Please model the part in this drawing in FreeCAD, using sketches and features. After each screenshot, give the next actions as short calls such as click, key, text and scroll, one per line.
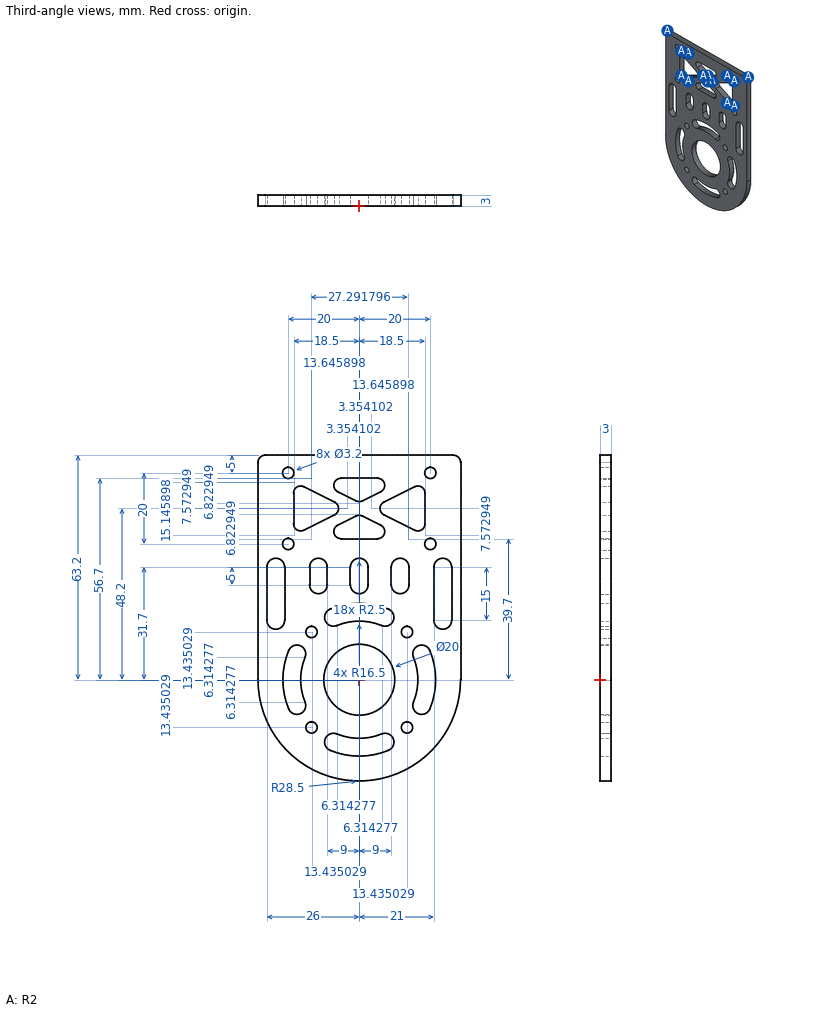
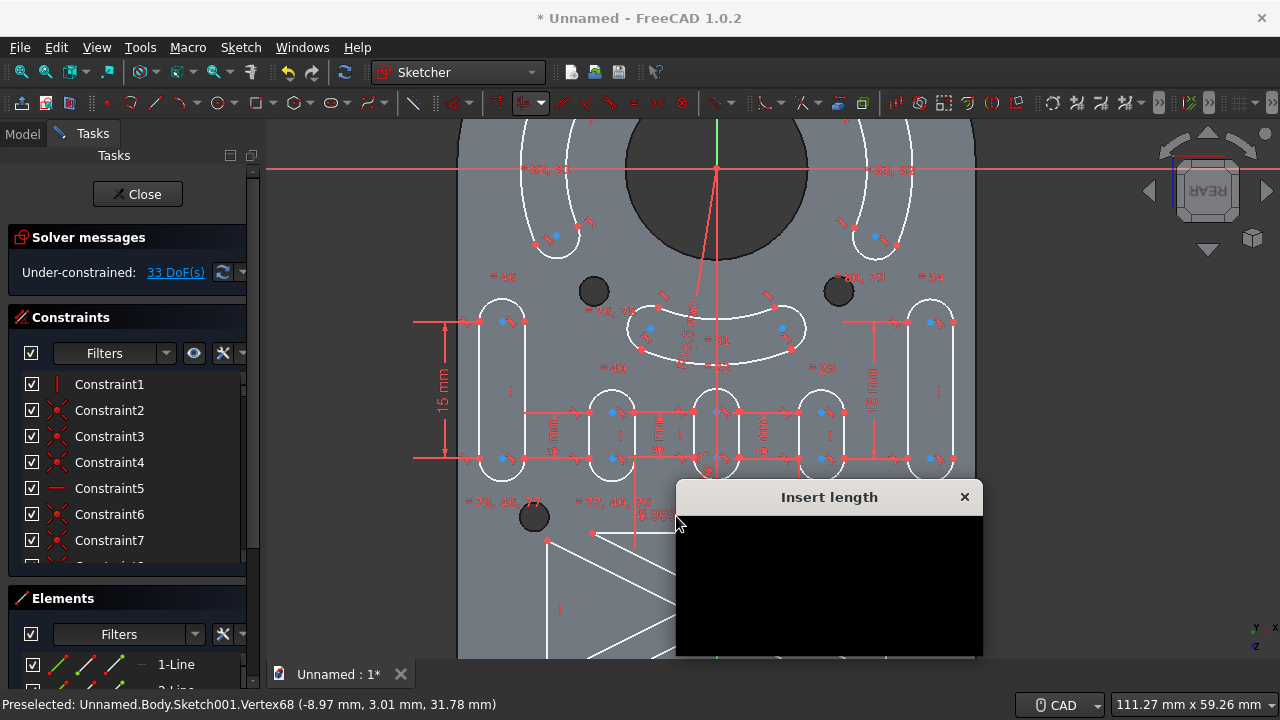
text(9)
key(Return)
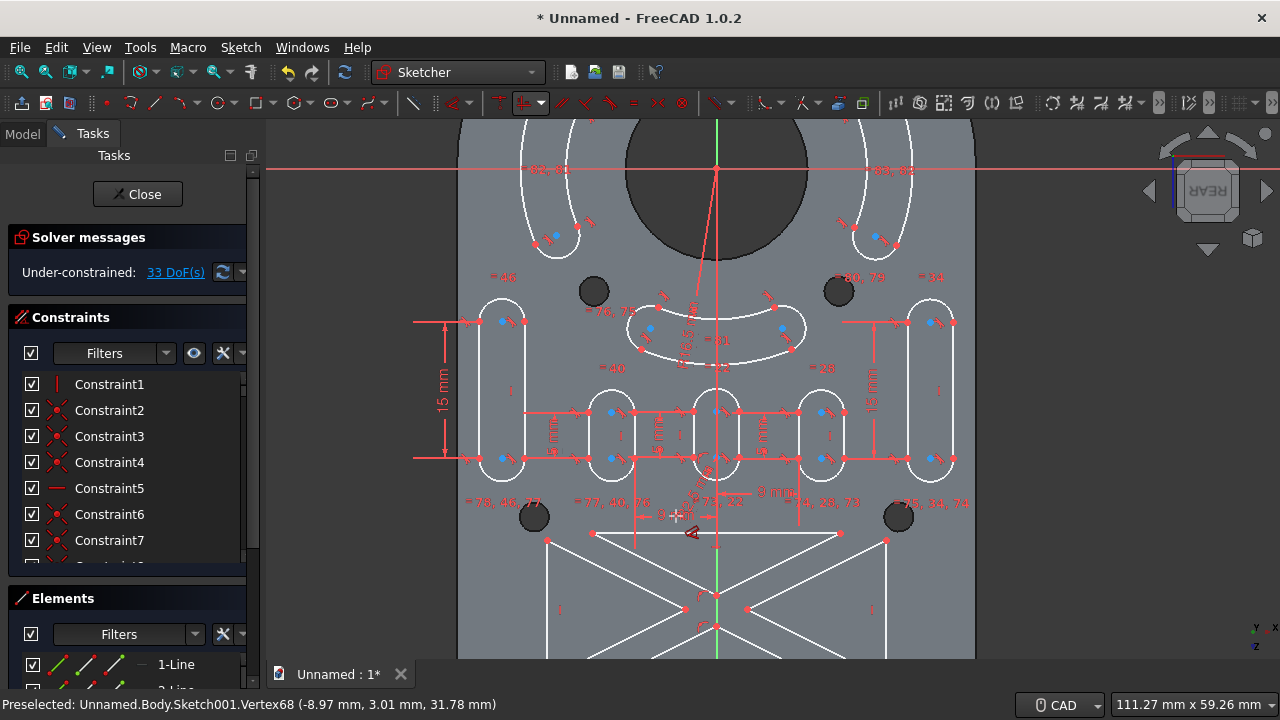
click(908, 459)
click(856, 493)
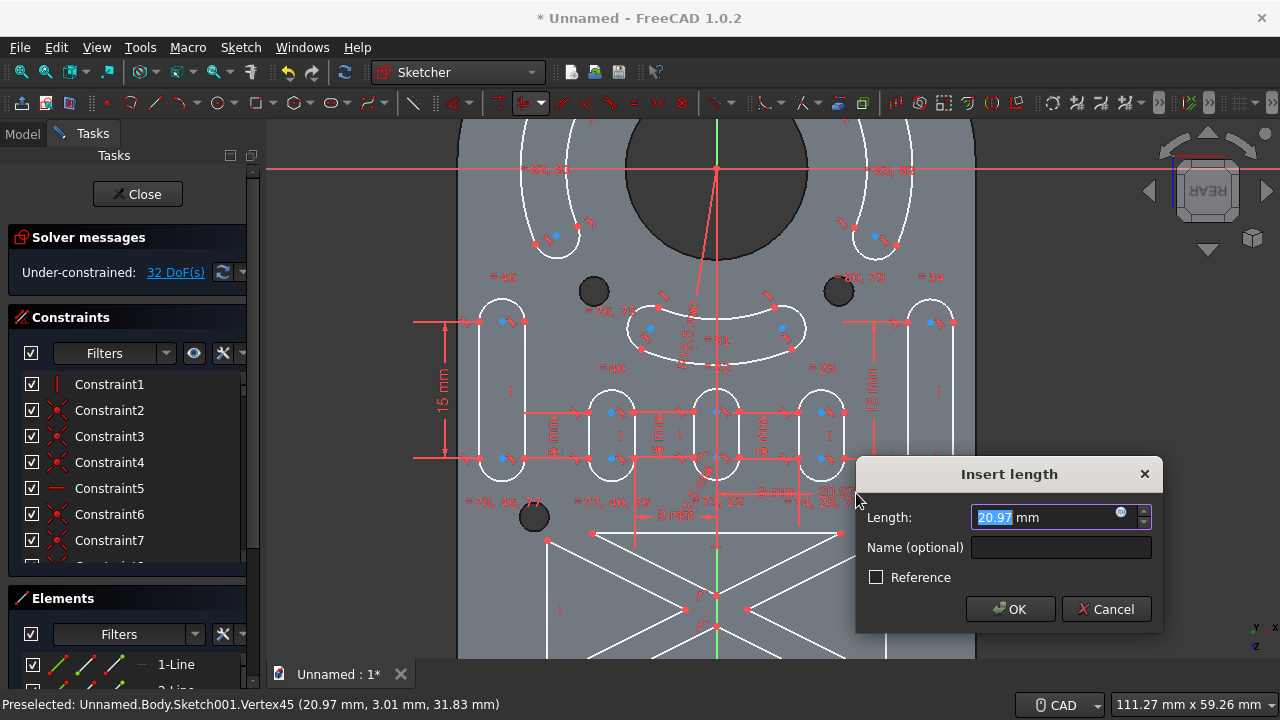
text(21)
key(Return)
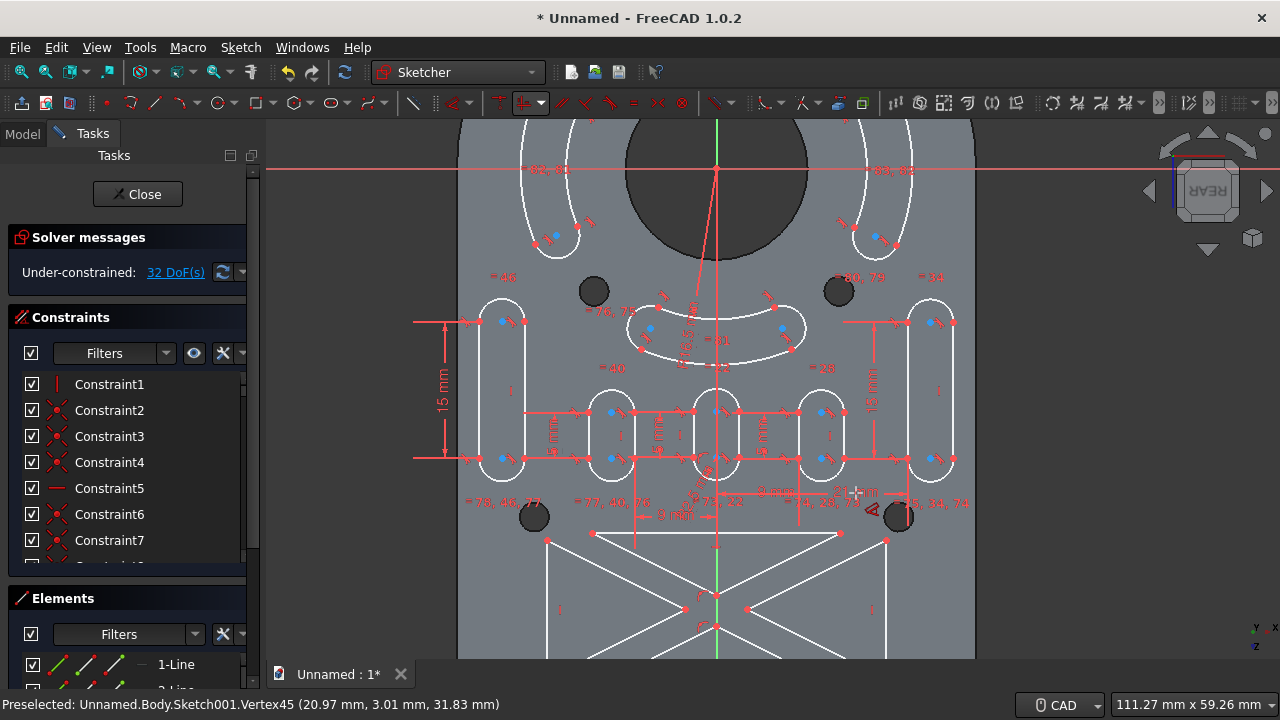
click(479, 458)
click(598, 492)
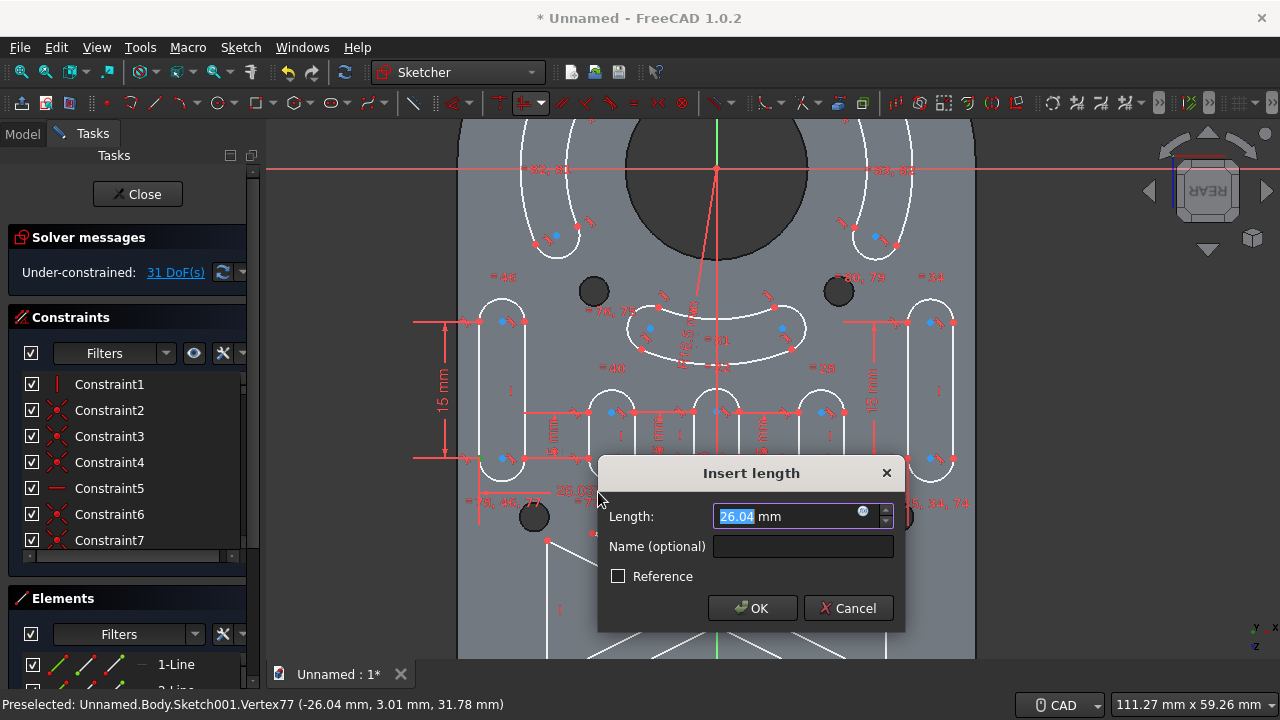
text(26)
key(Return)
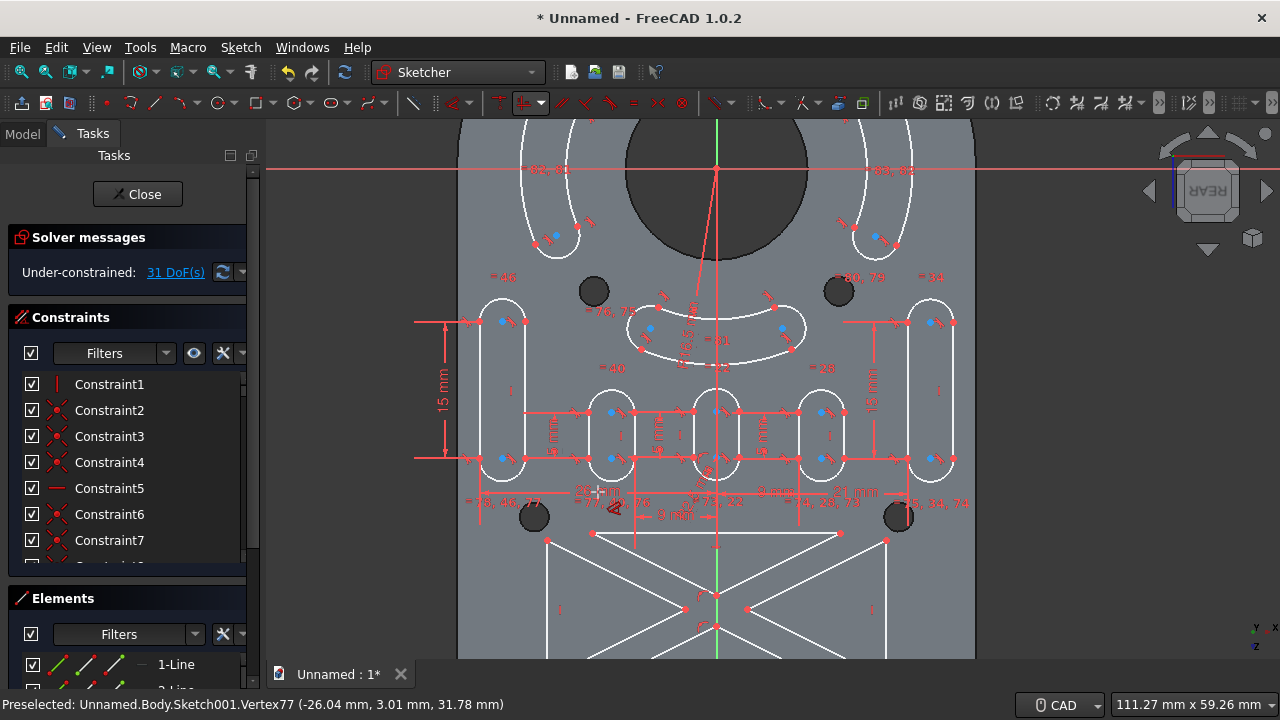
click(547, 540)
click(573, 574)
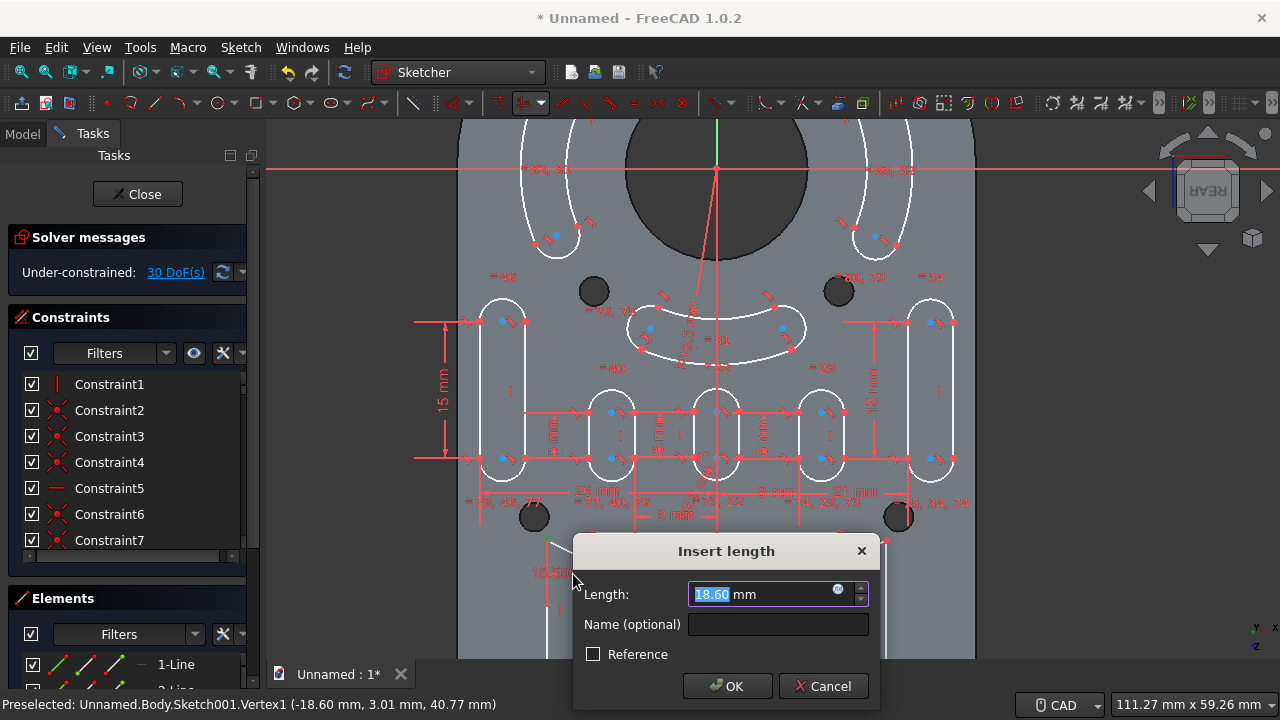
text(18.5)
key(Return)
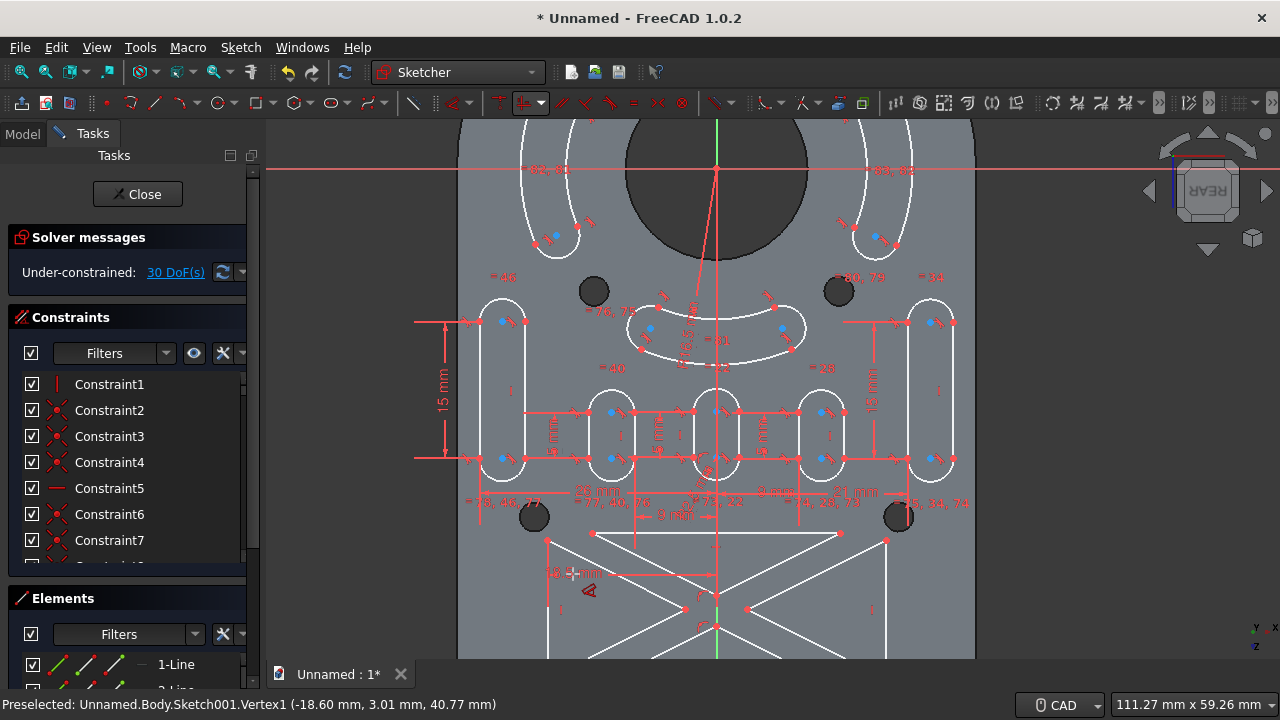
click(686, 610)
click(652, 389)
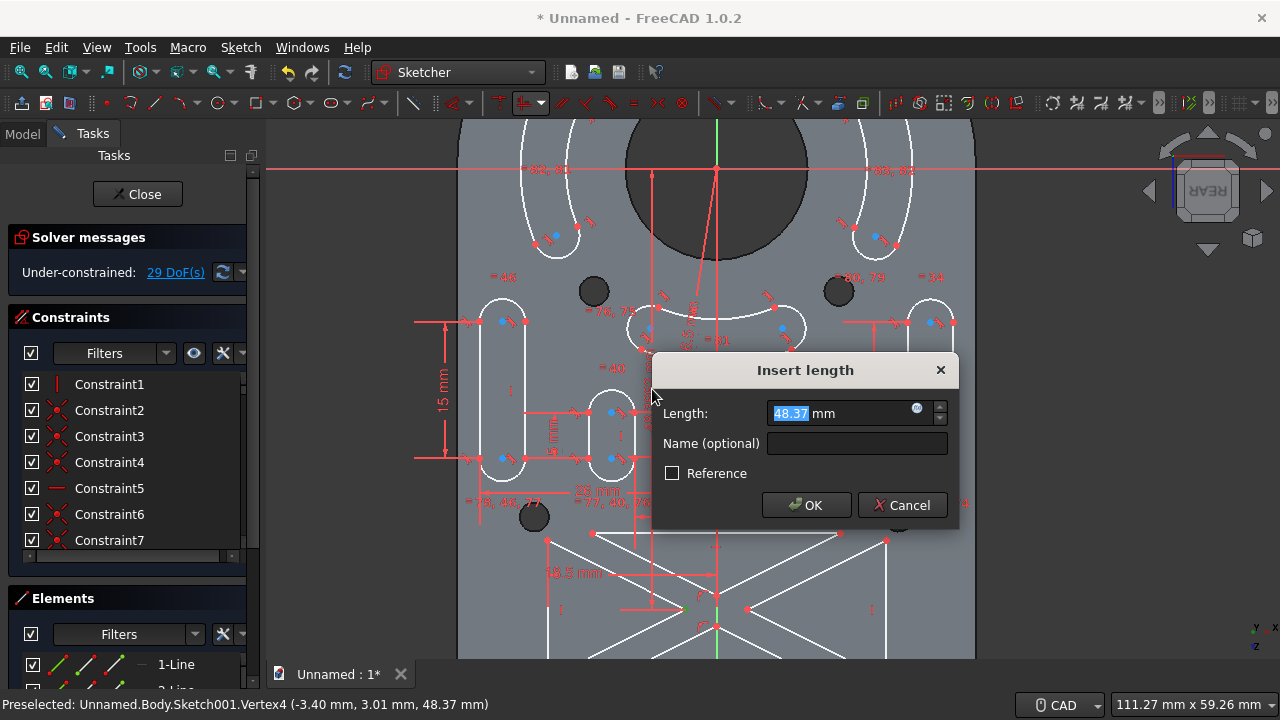
text(48.2)
key(Return)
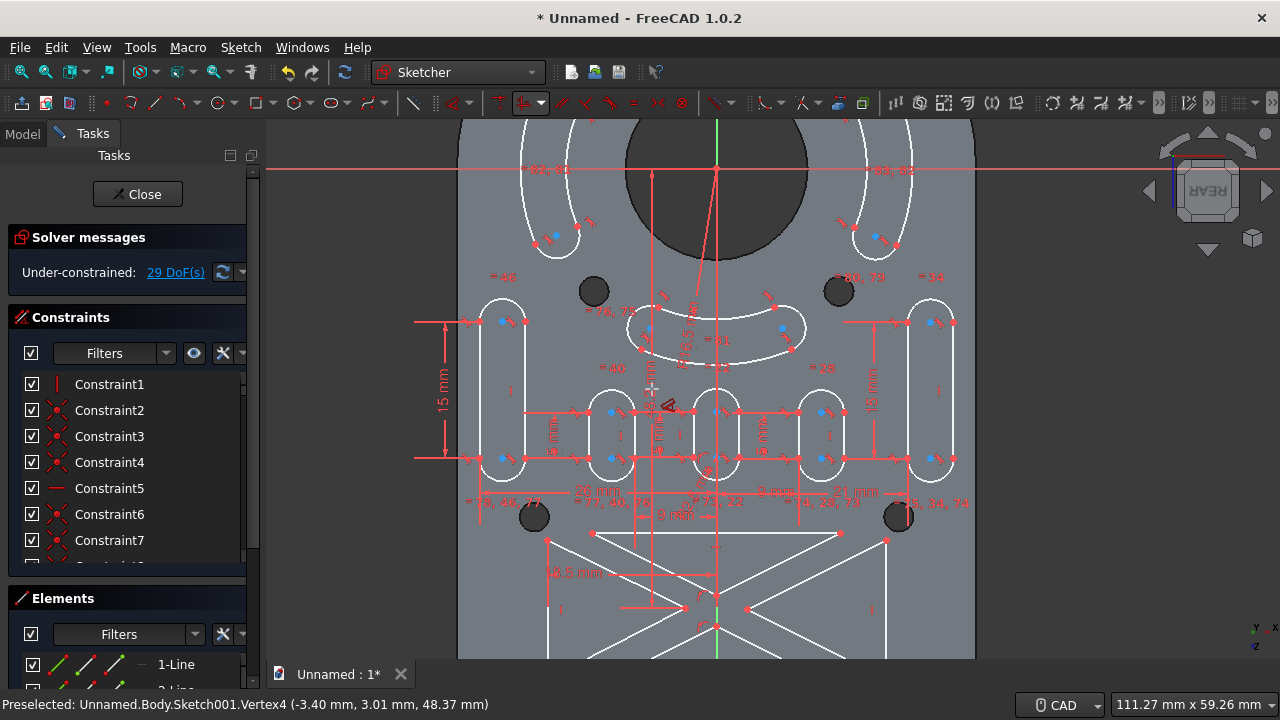
click(840, 533)
click(874, 351)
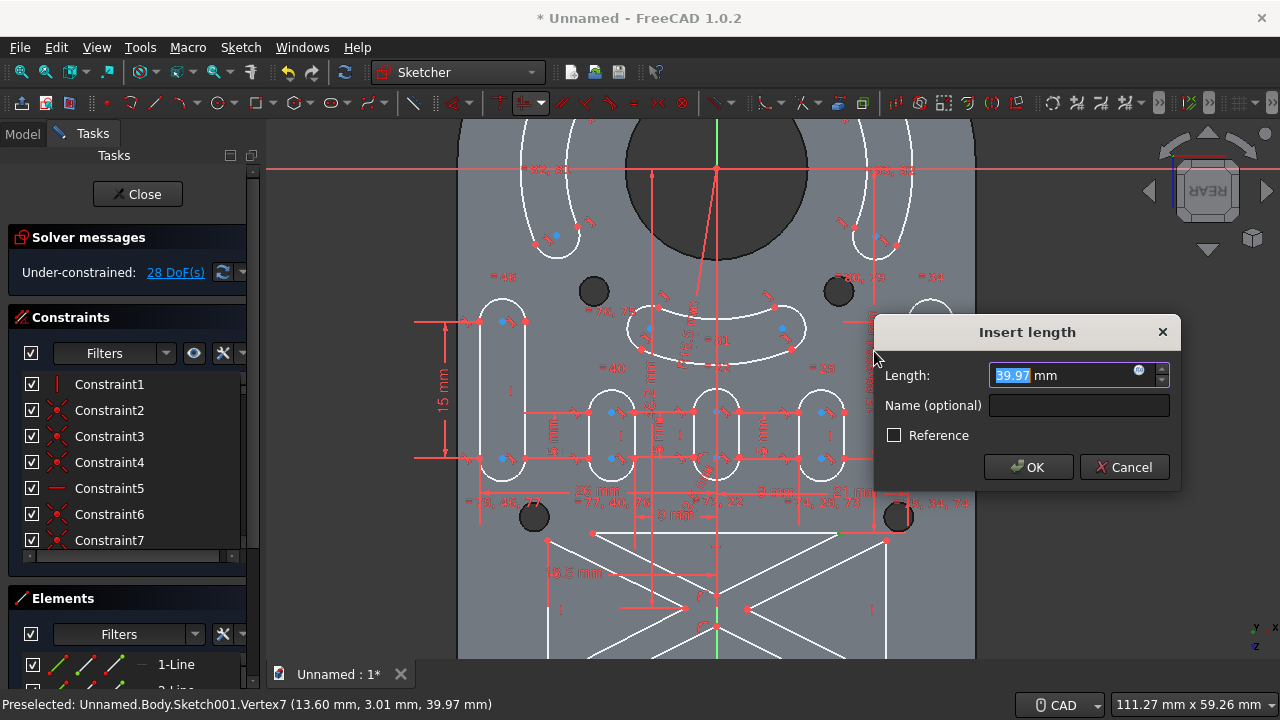
text(39.7)
key(Return)